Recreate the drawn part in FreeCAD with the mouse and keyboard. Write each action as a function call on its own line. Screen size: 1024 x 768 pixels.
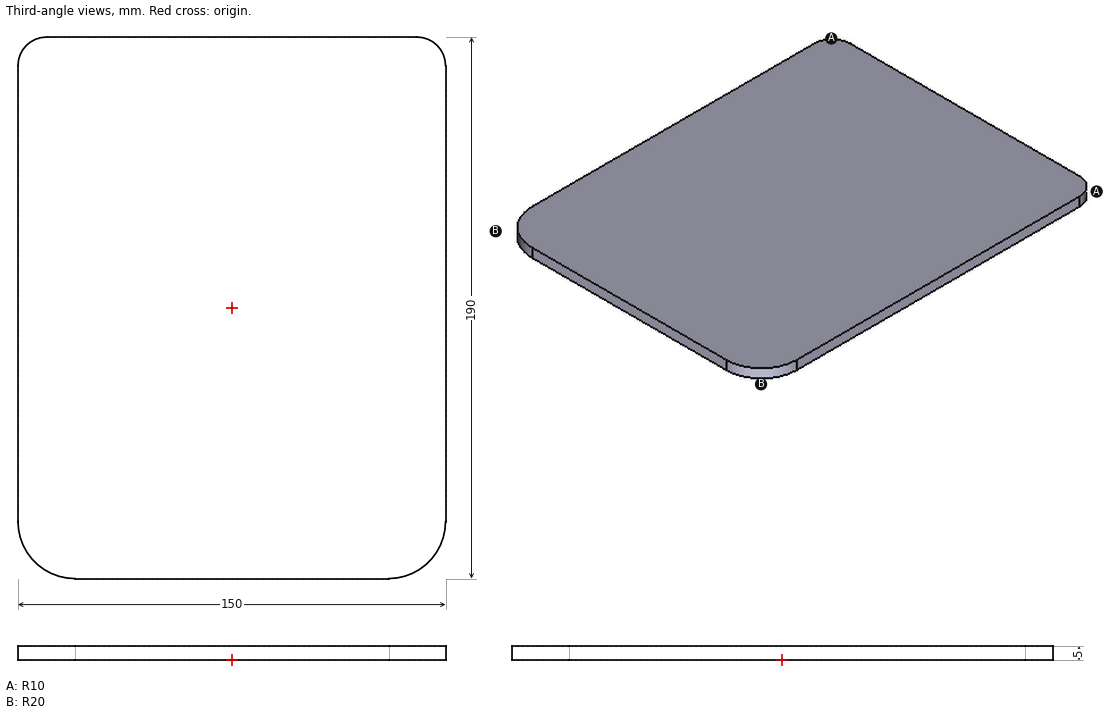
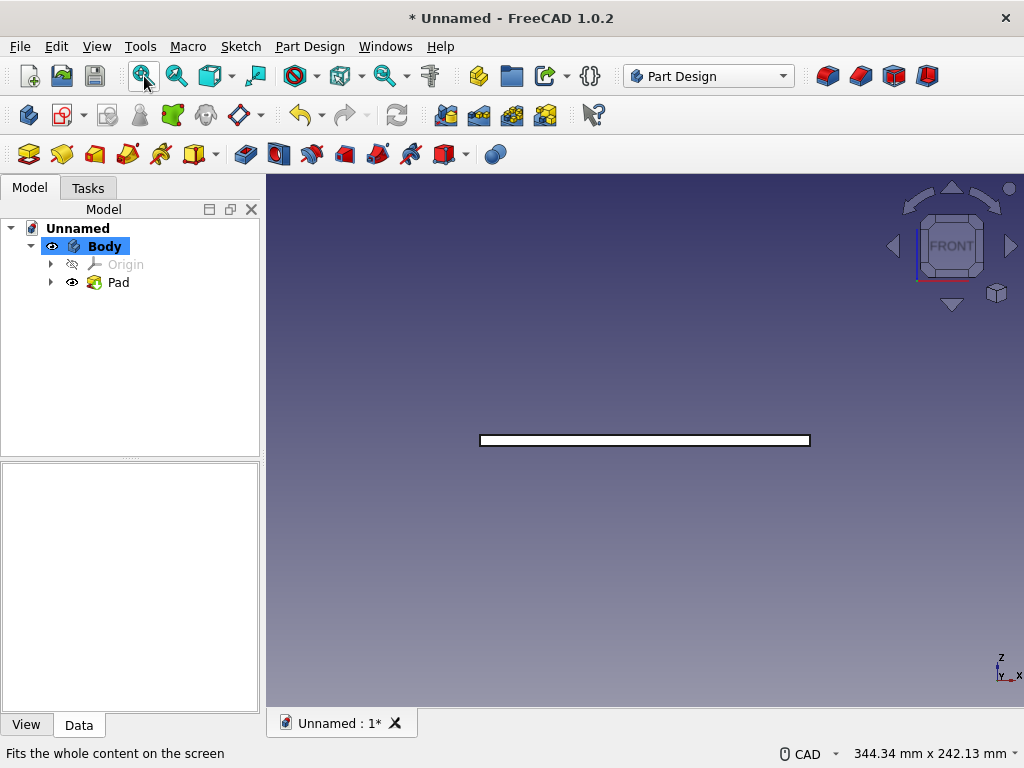
click(144, 76)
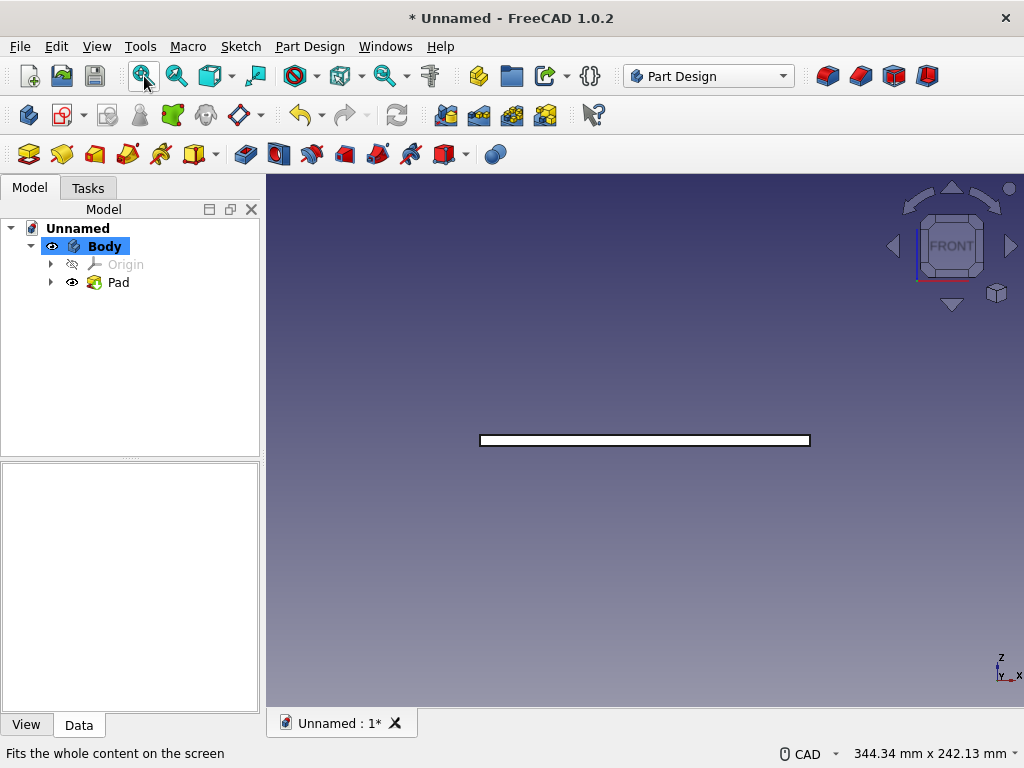
scroll(480, 440, up, 7)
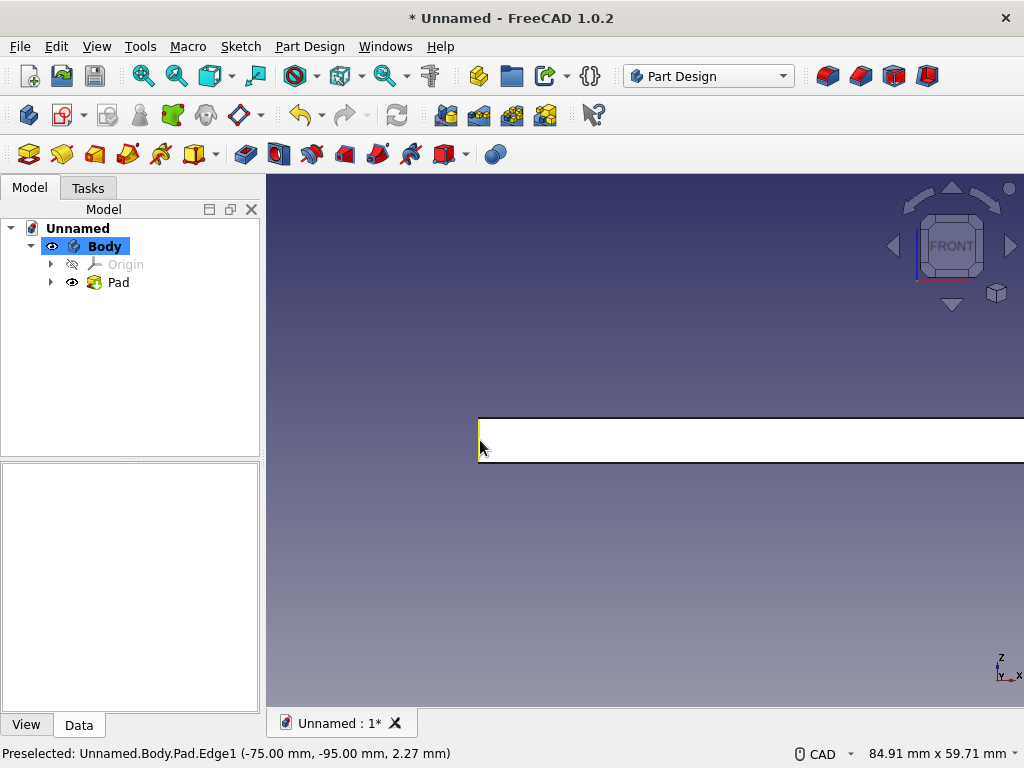
click(144, 76)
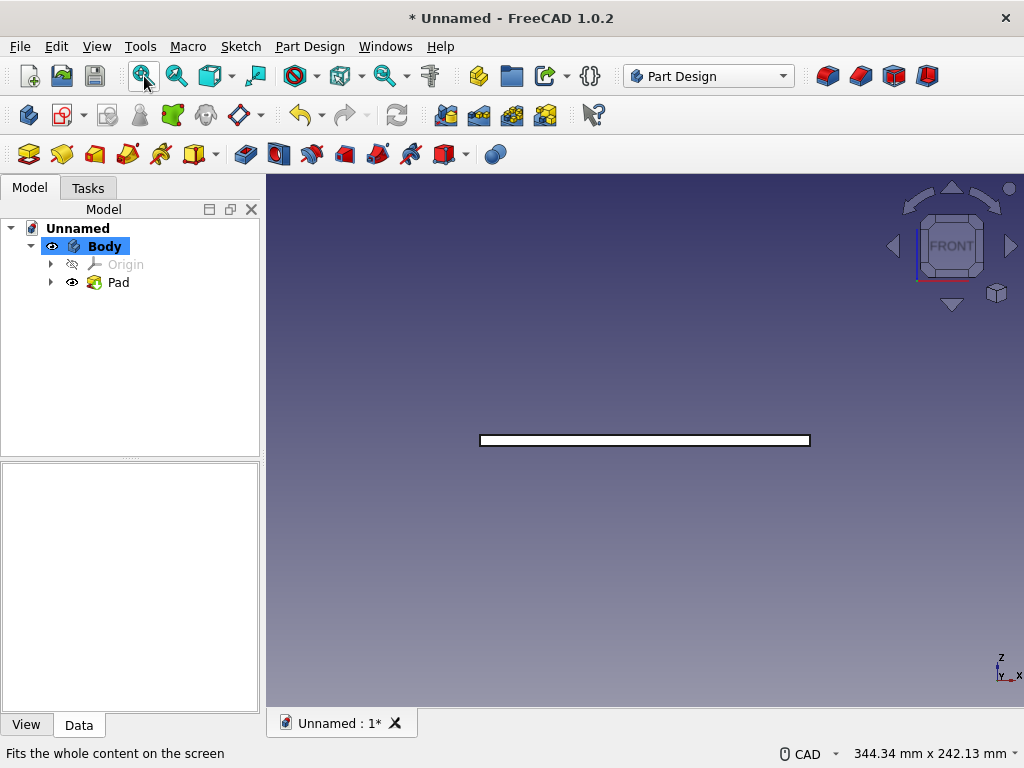
key(3)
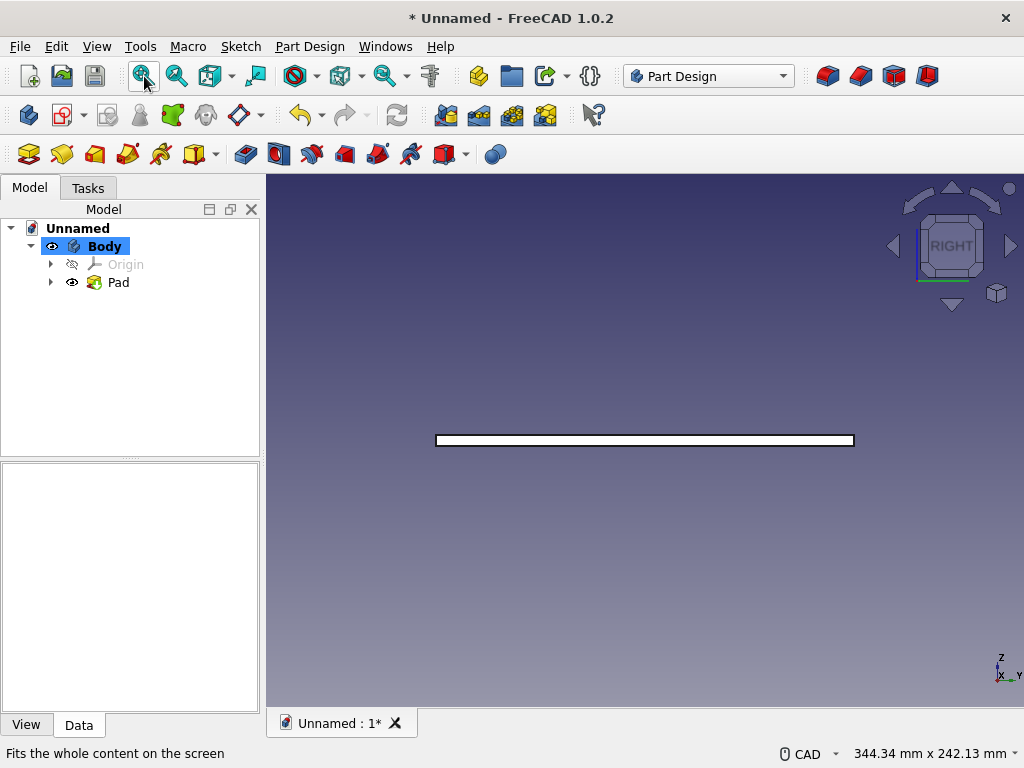
scroll(854, 439, up, 7)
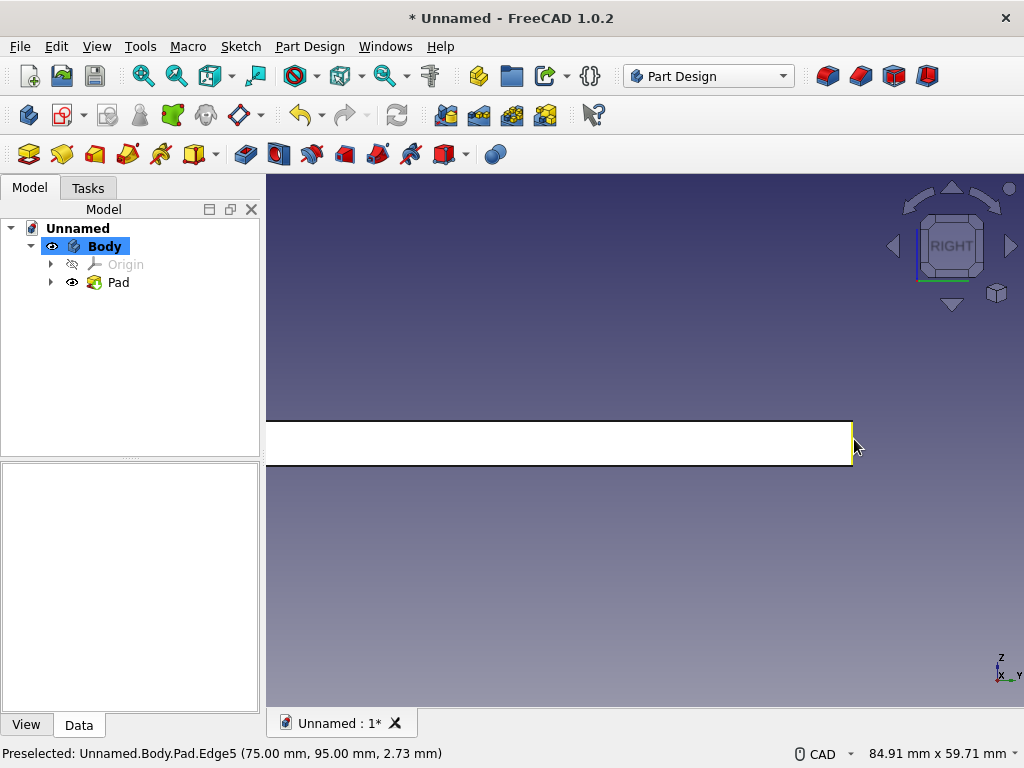
click(852, 443)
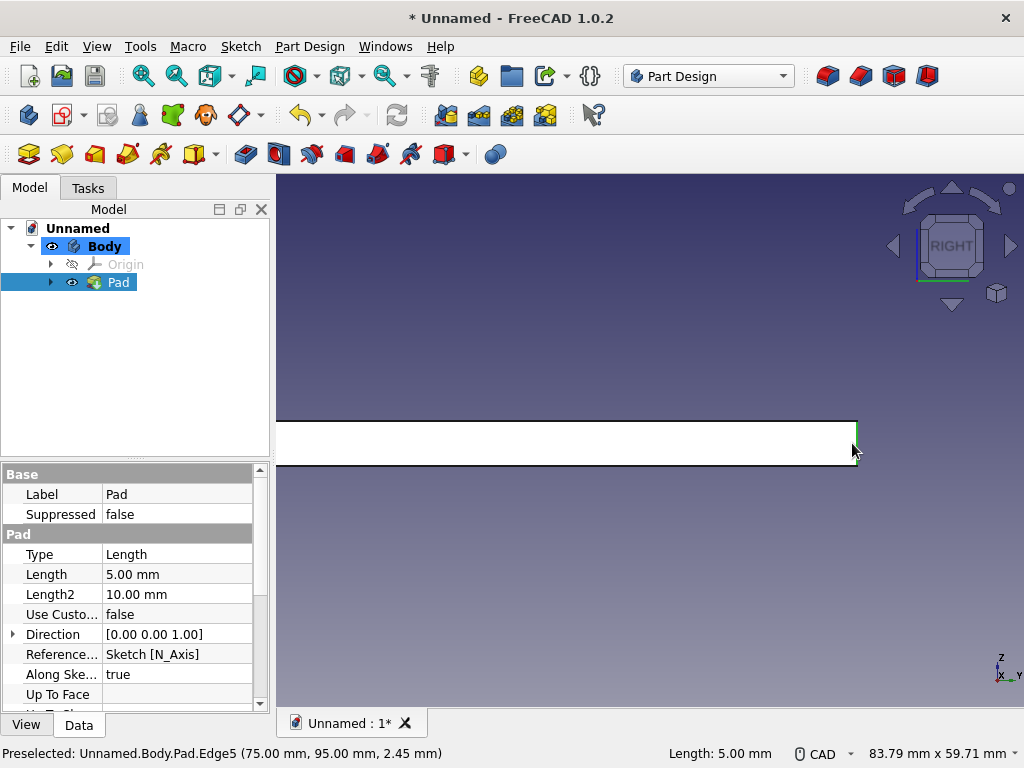
click(144, 76)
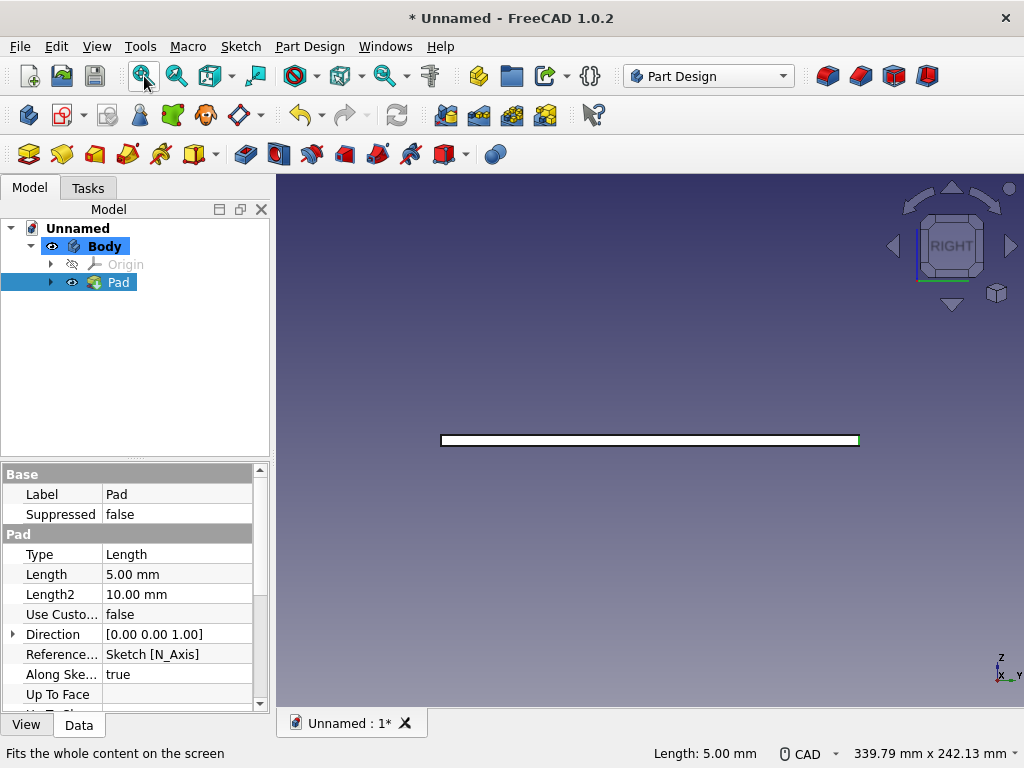
key(5)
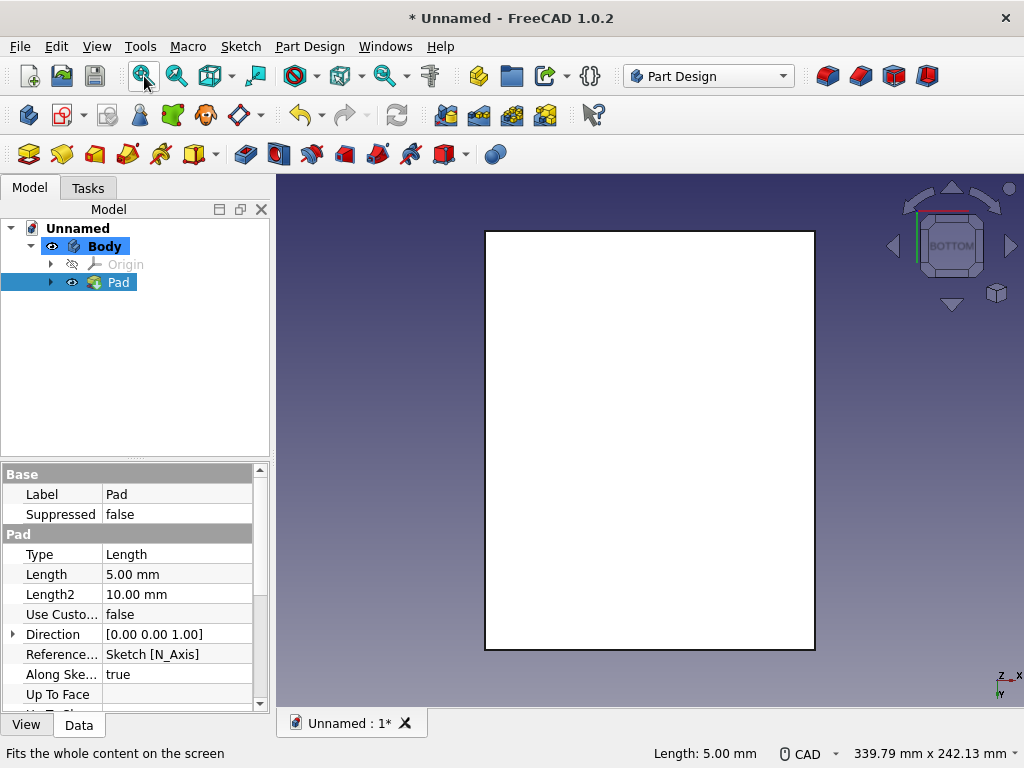
scroll(485, 649, up, 7)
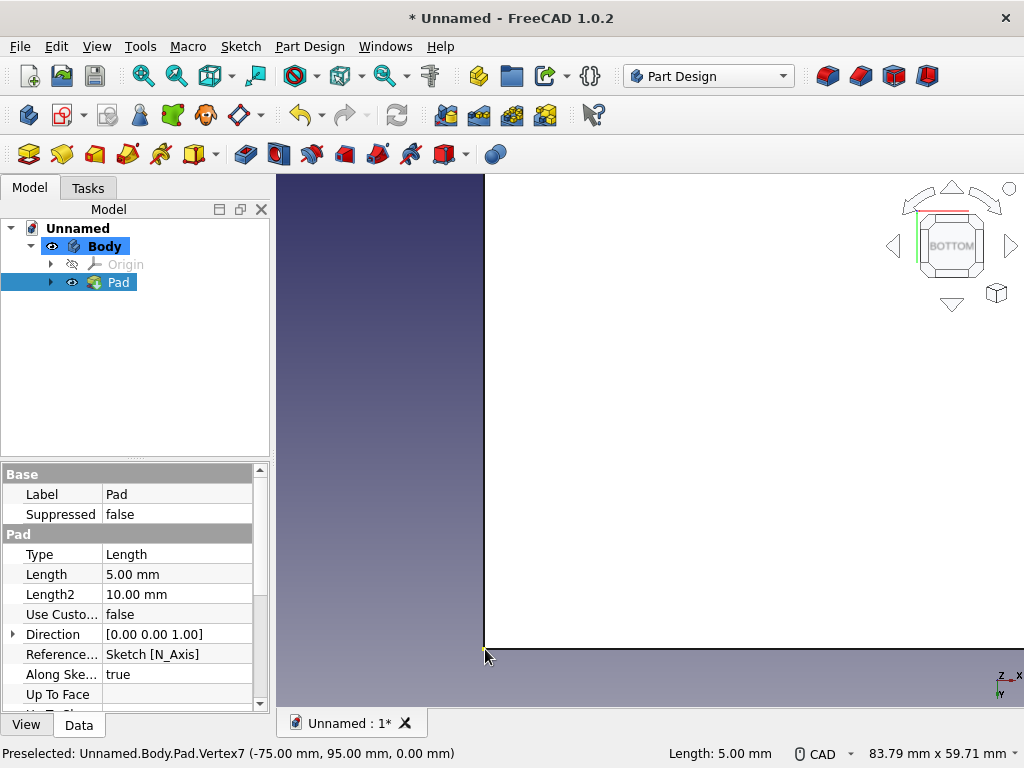
click(144, 76)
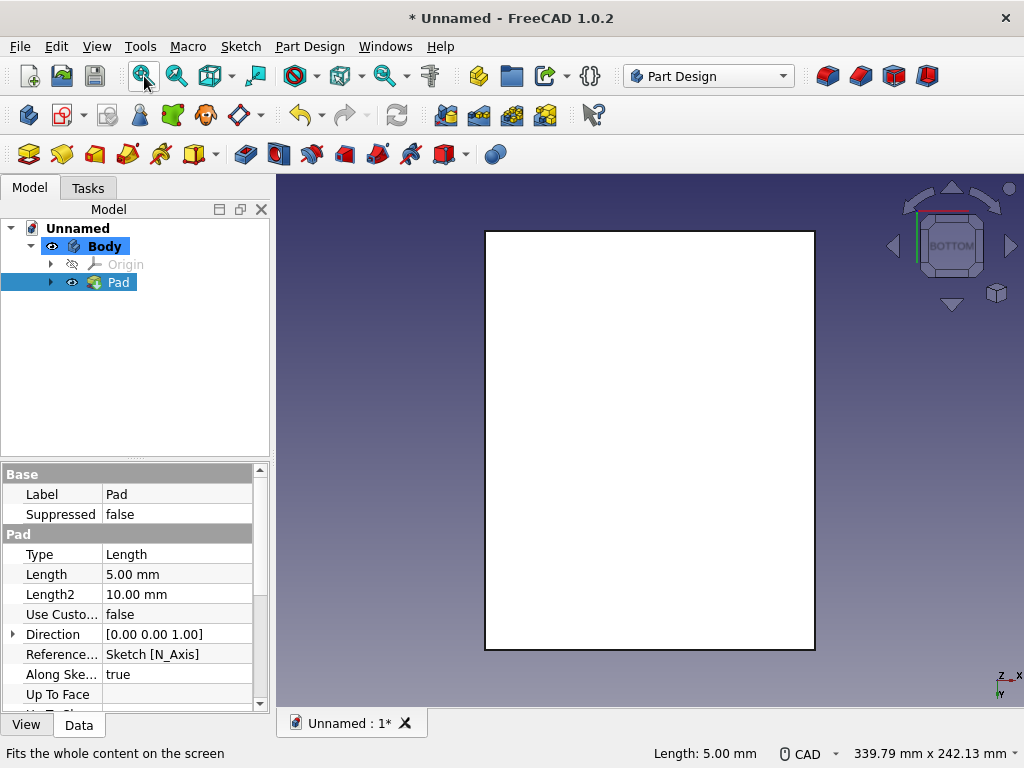
key(4)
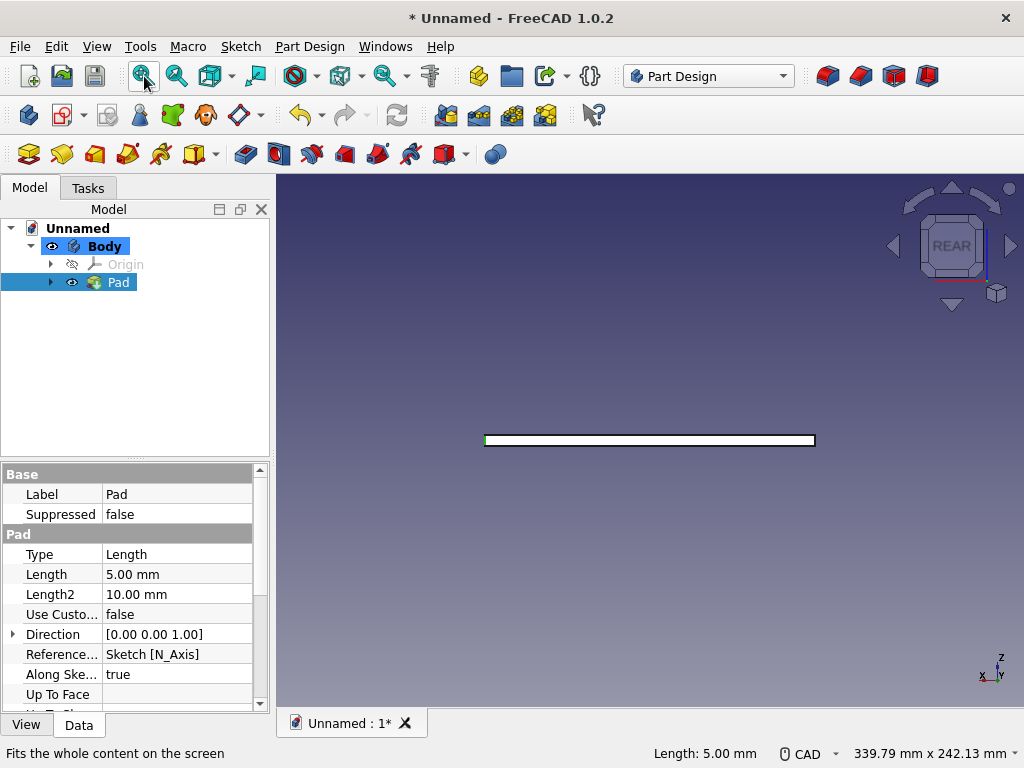
click(144, 76)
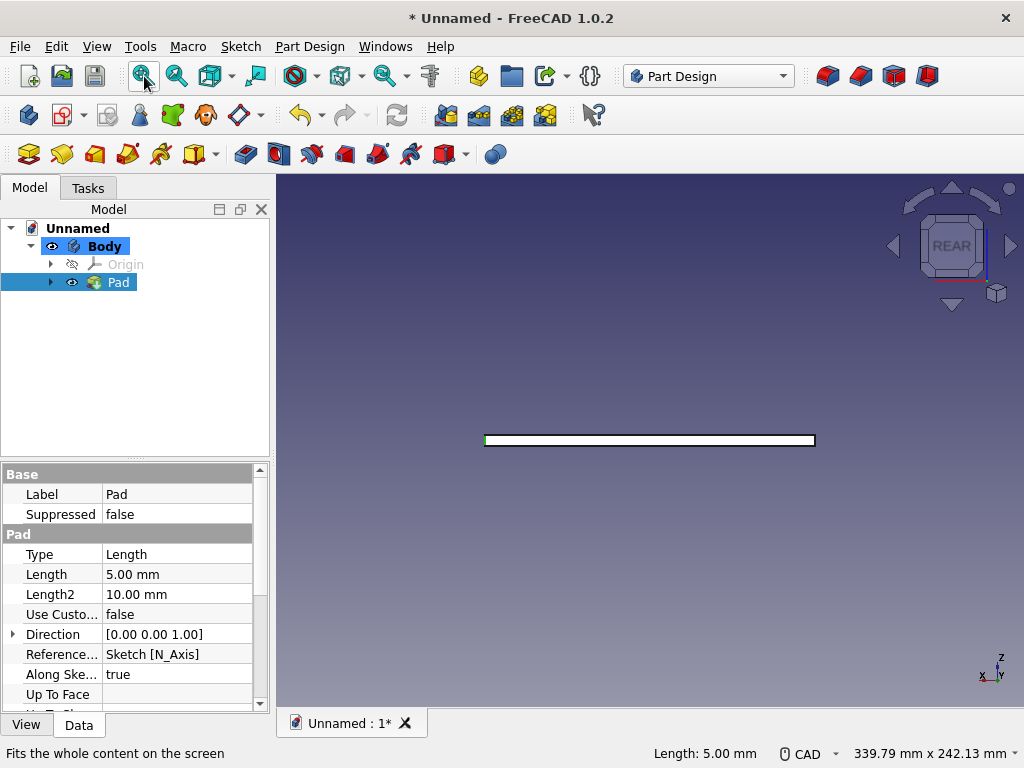
scroll(815, 440, up, 7)